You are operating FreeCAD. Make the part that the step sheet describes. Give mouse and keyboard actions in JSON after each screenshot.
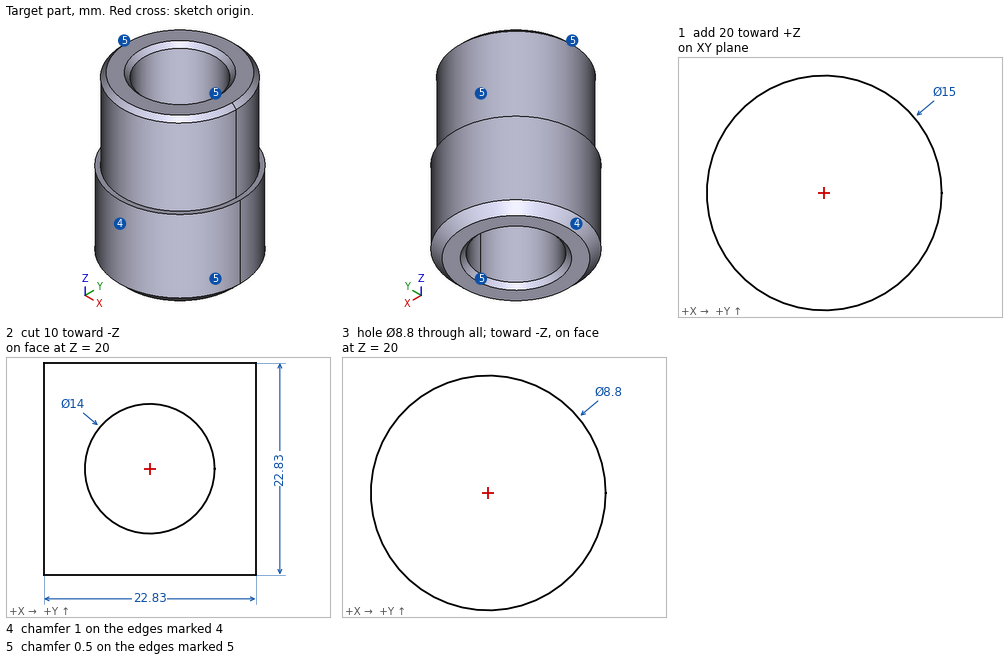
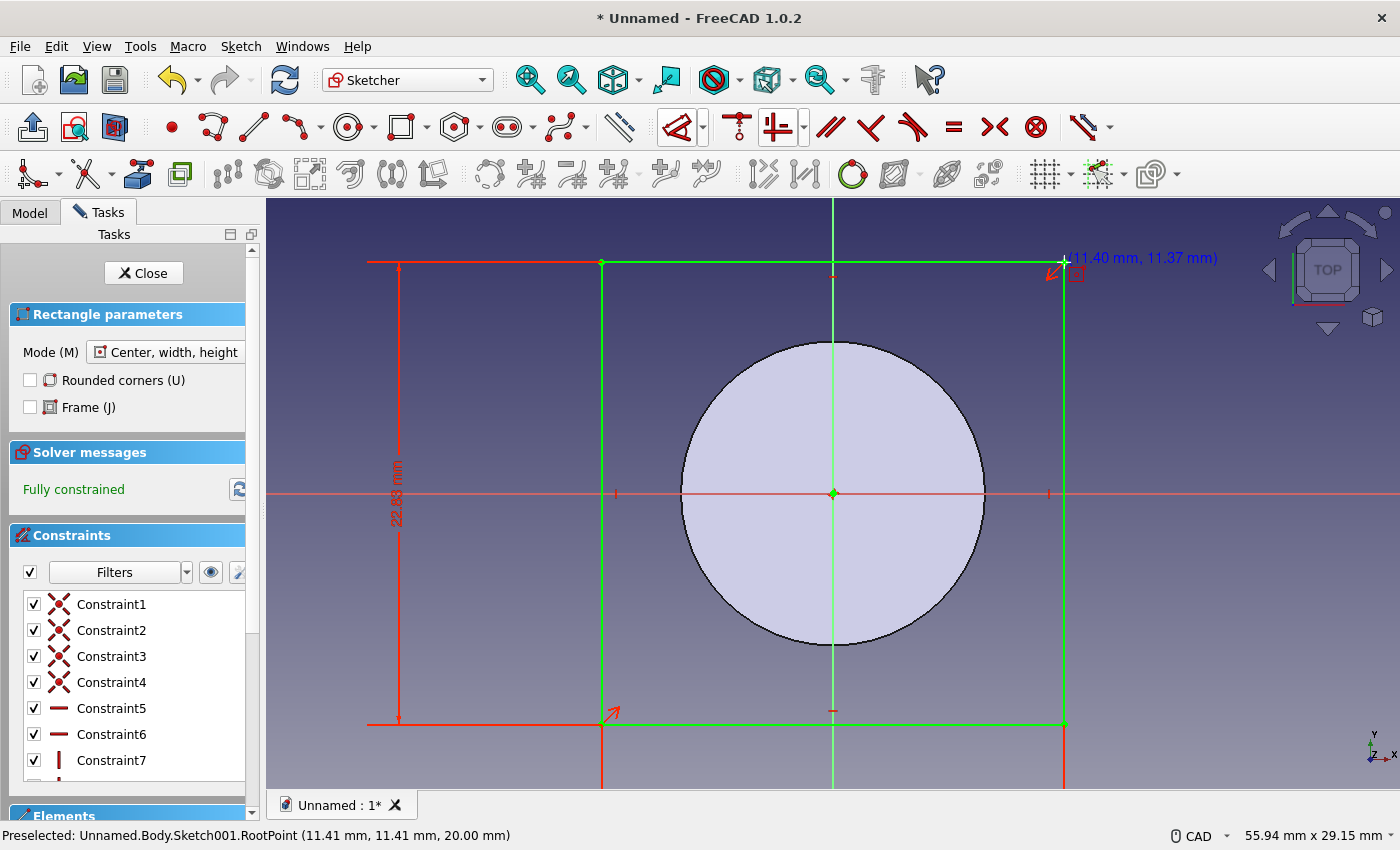
{"action": "left_click", "coordinate": [348, 128]}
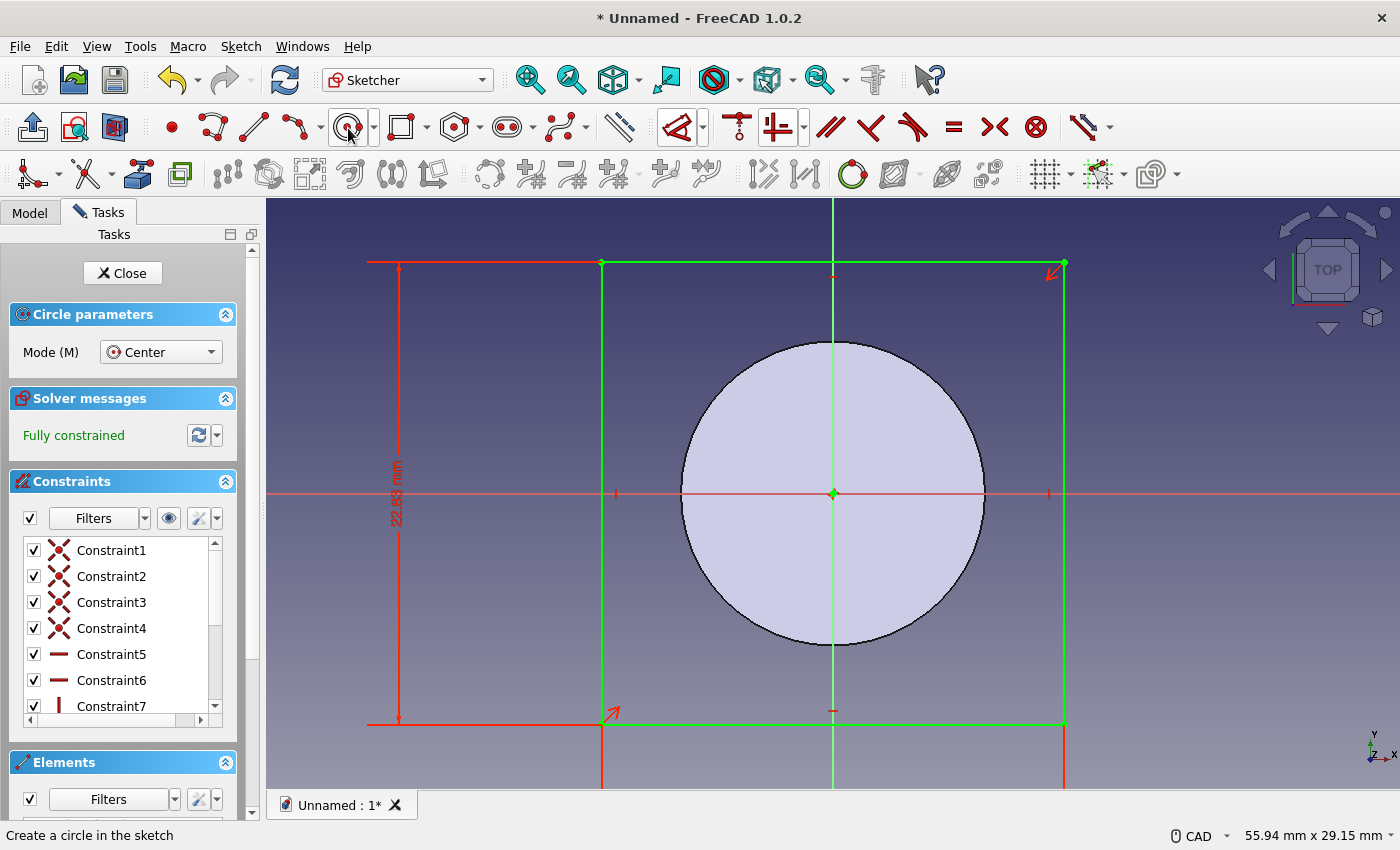
{"action": "left_click", "coordinate": [833, 494]}
{"action": "mouse_move", "coordinate": [933, 393]}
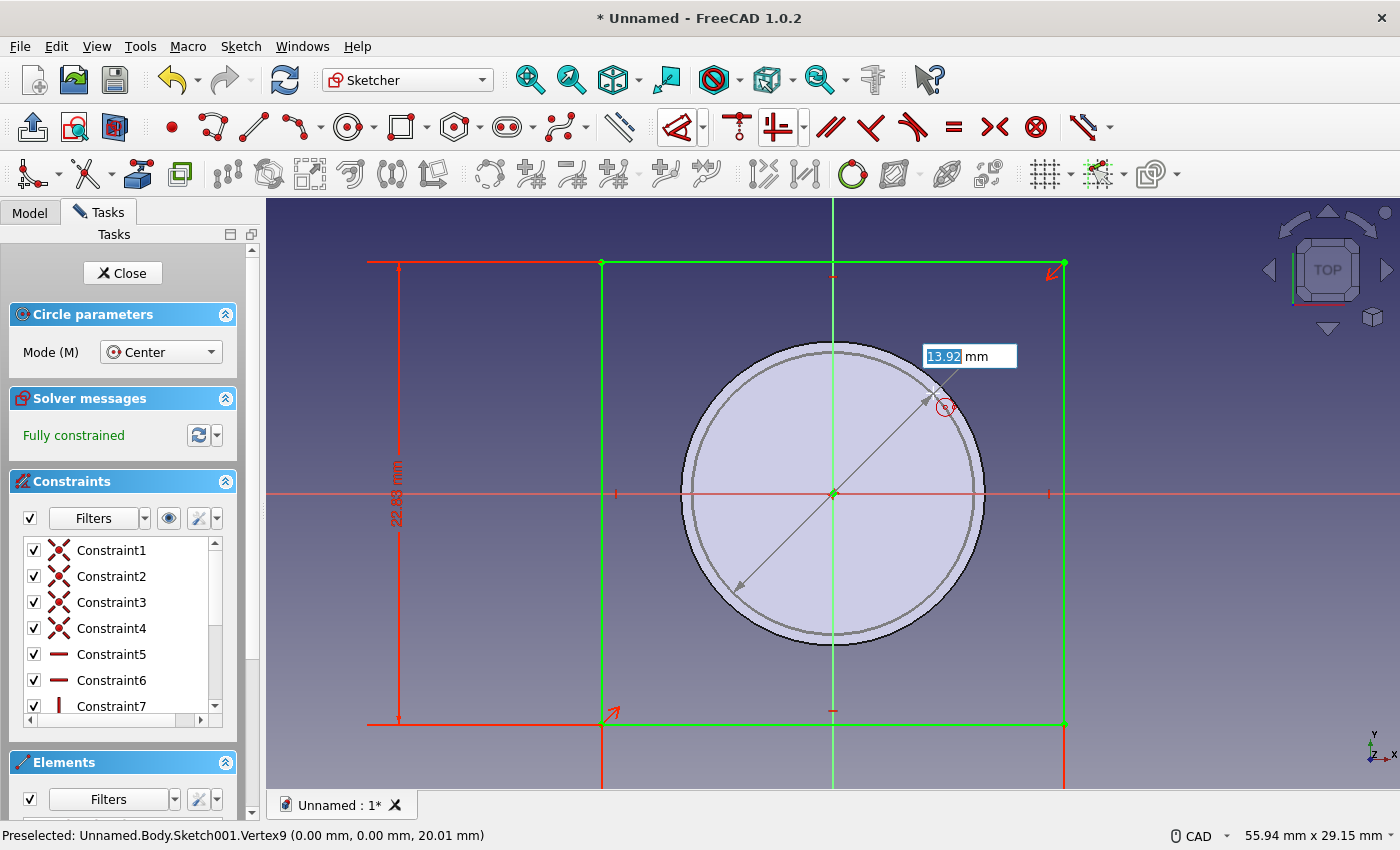
{"action": "type", "text": "14"}
{"action": "key", "text": "Return"}
{"action": "key", "text": "Escape"}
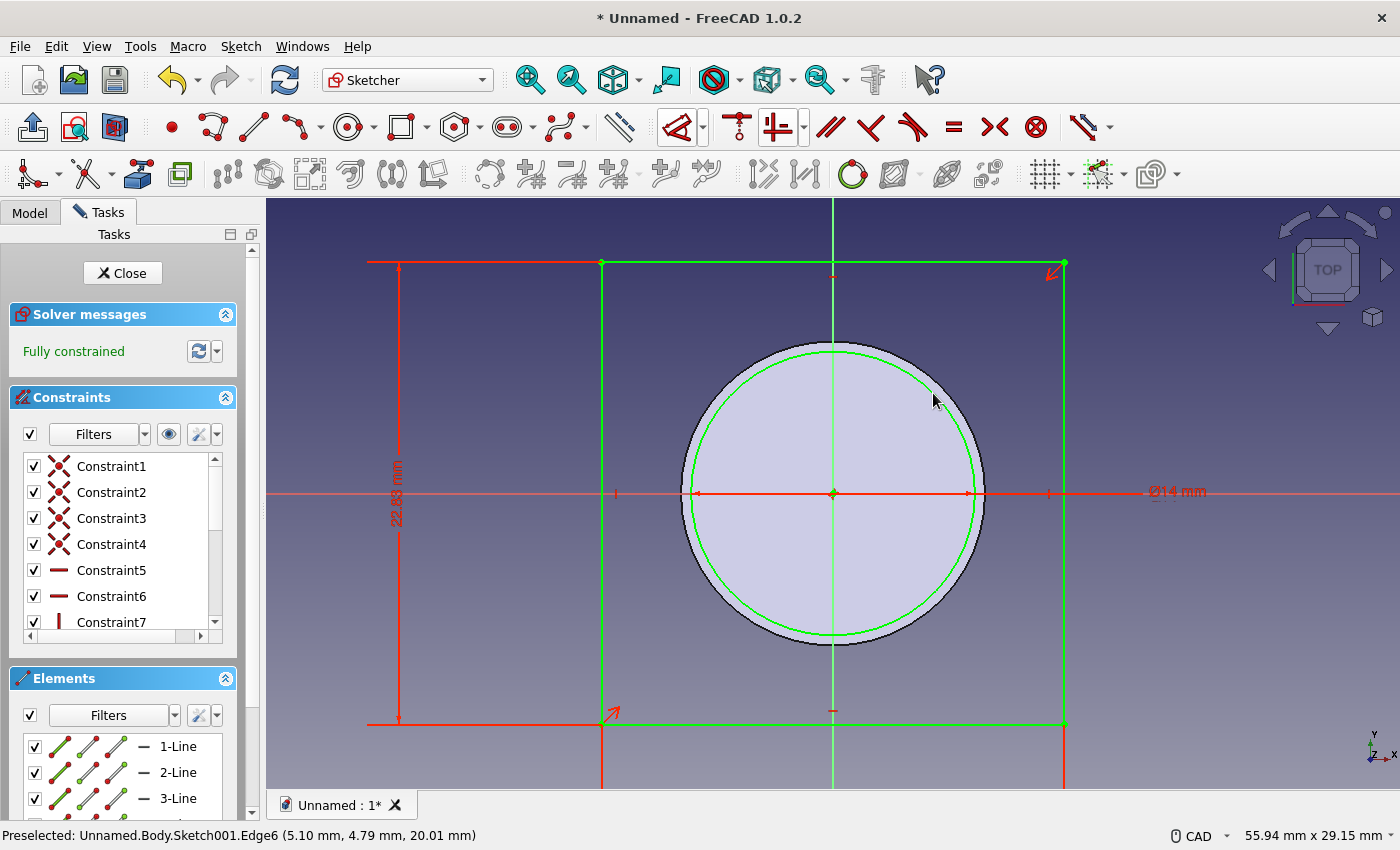
{"action": "left_click", "coordinate": [123, 273]}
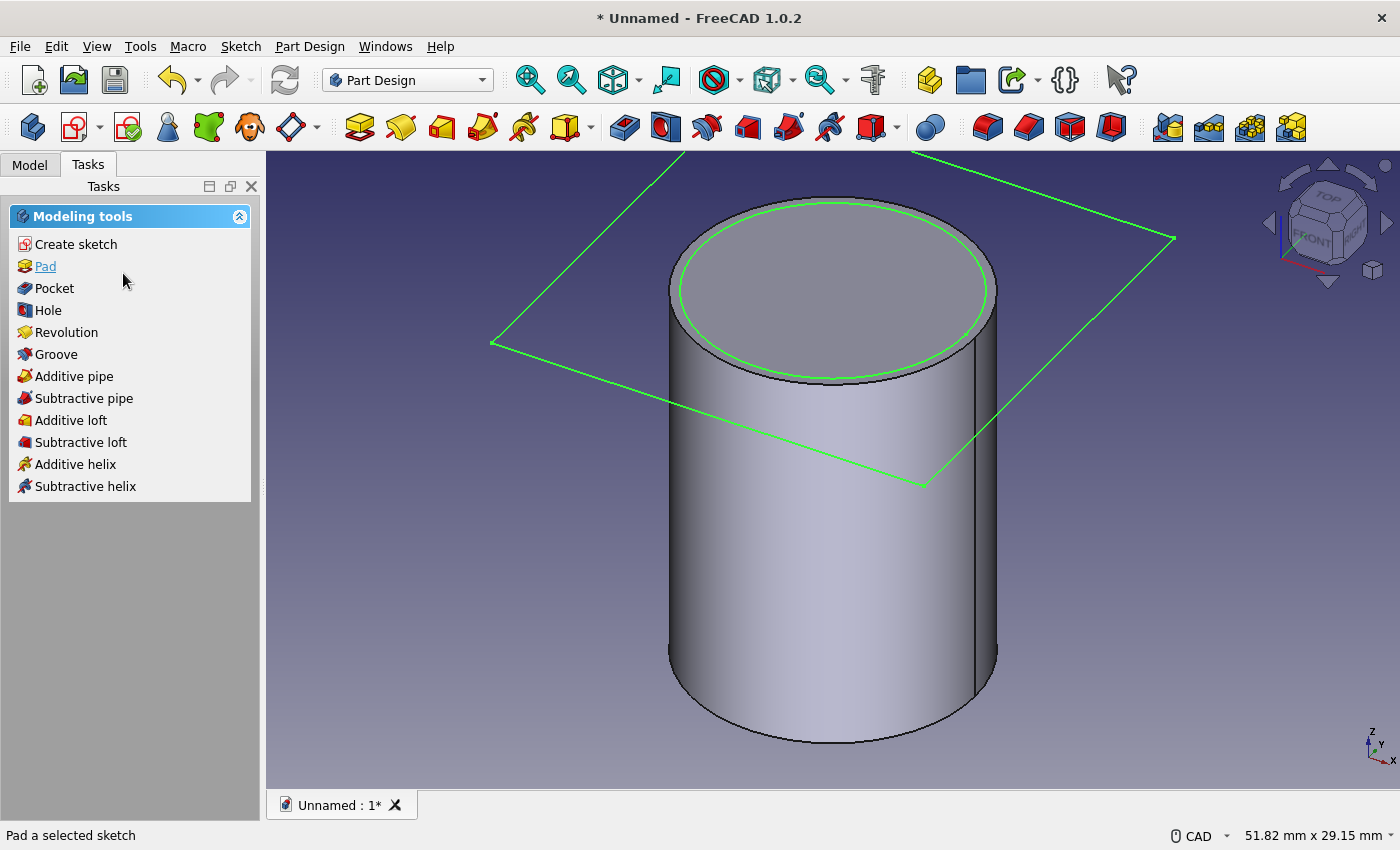
{"action": "left_click", "coordinate": [625, 128]}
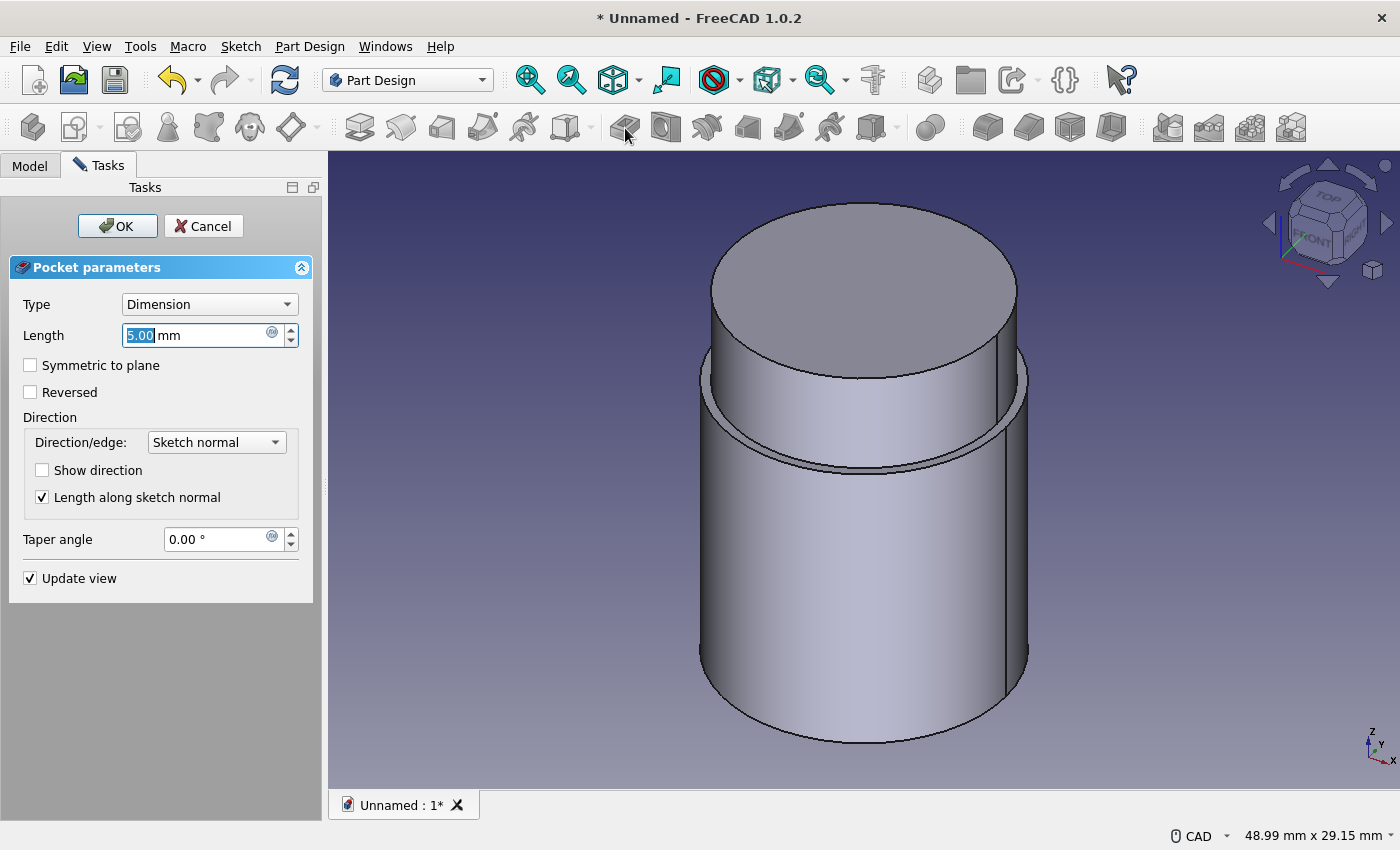
{"action": "type", "text": "10"}
{"action": "key", "text": "Tab"}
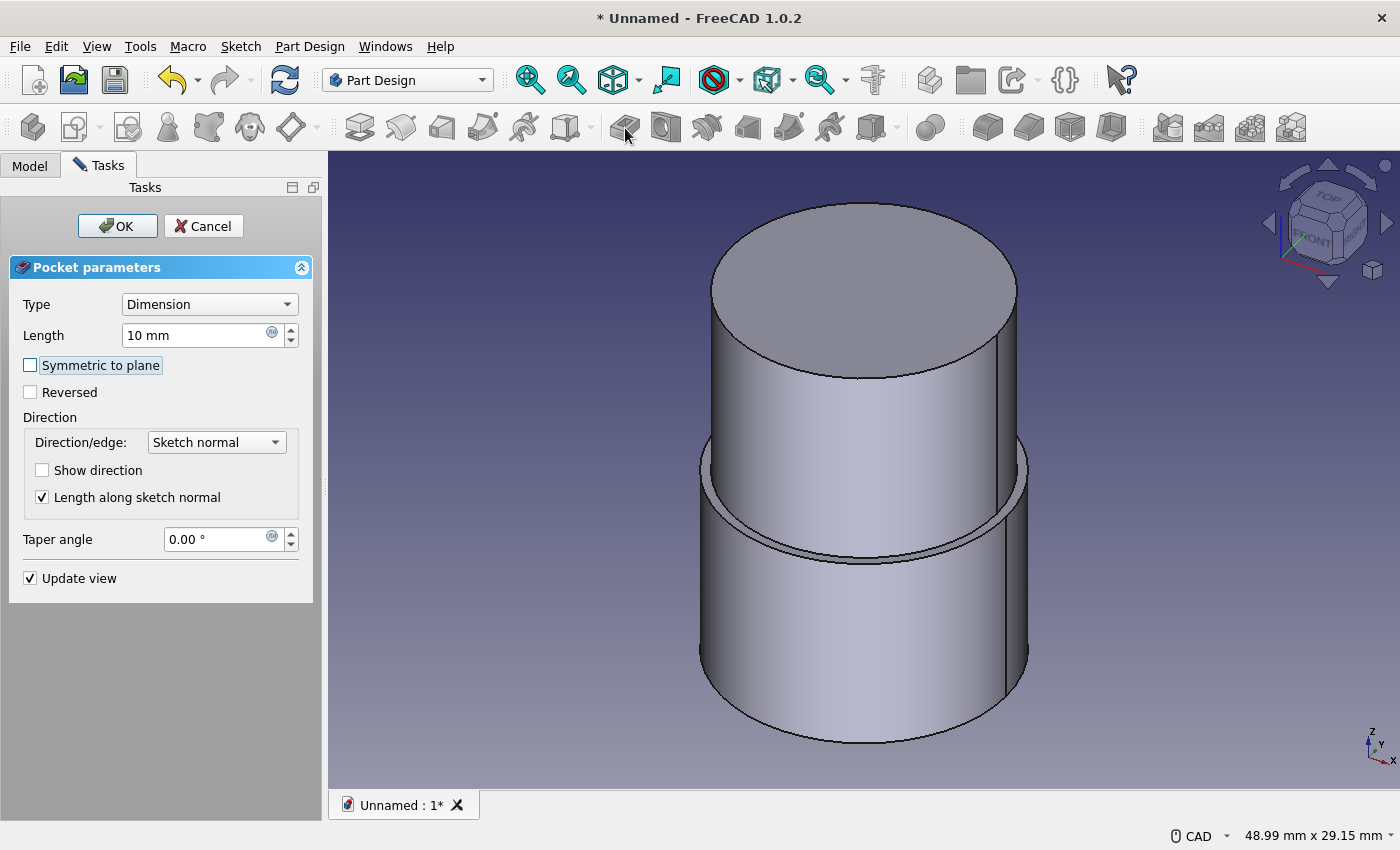
{"action": "left_click", "coordinate": [118, 226]}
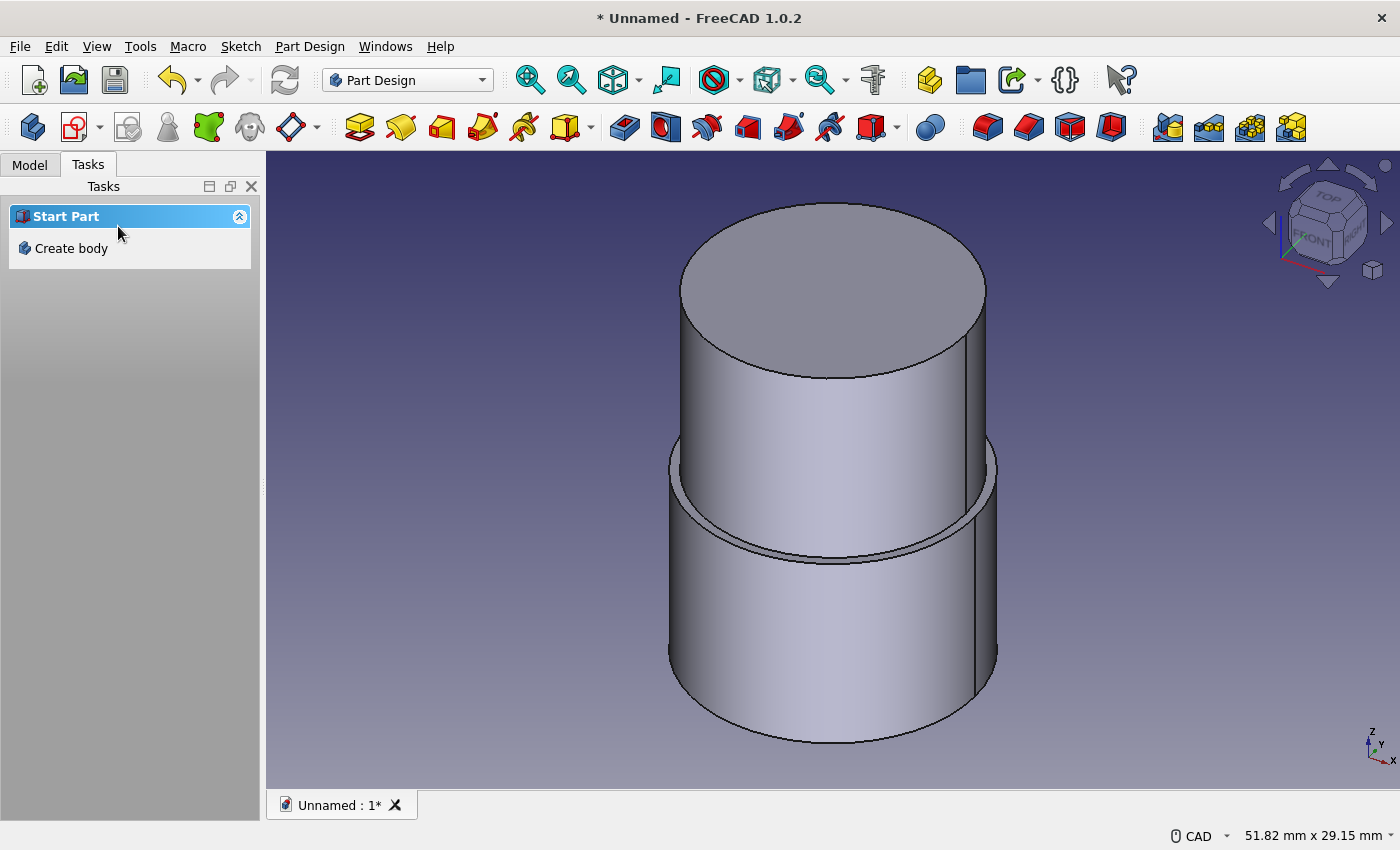
{"action": "left_click", "coordinate": [833, 290]}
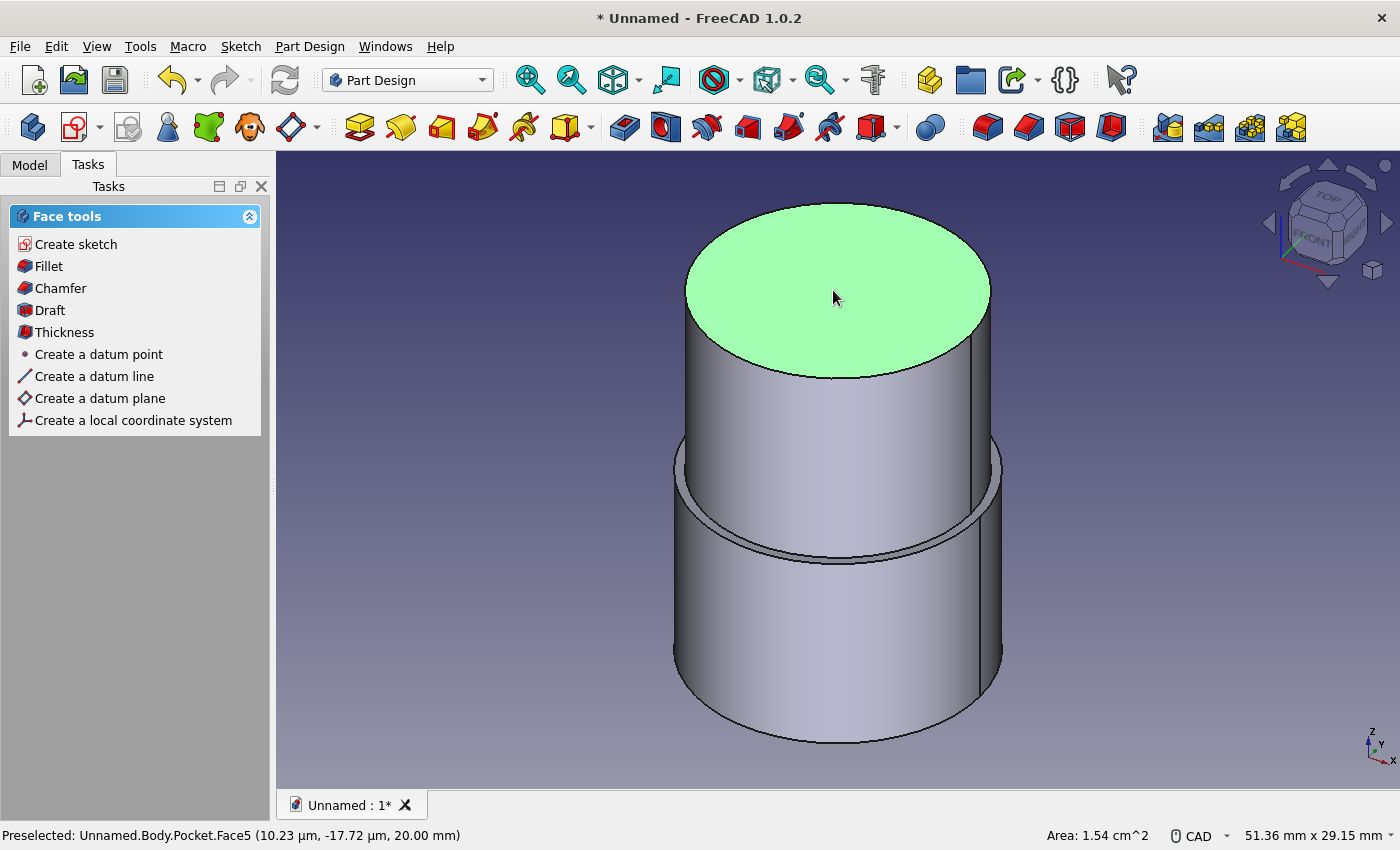
{"action": "left_click", "coordinate": [74, 128]}